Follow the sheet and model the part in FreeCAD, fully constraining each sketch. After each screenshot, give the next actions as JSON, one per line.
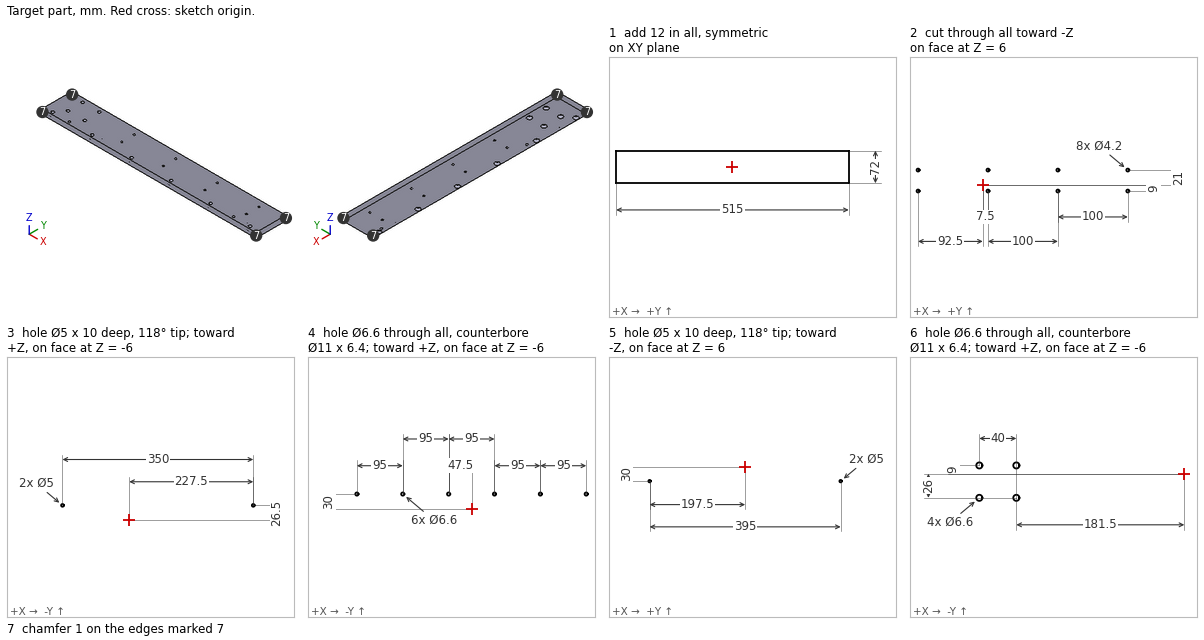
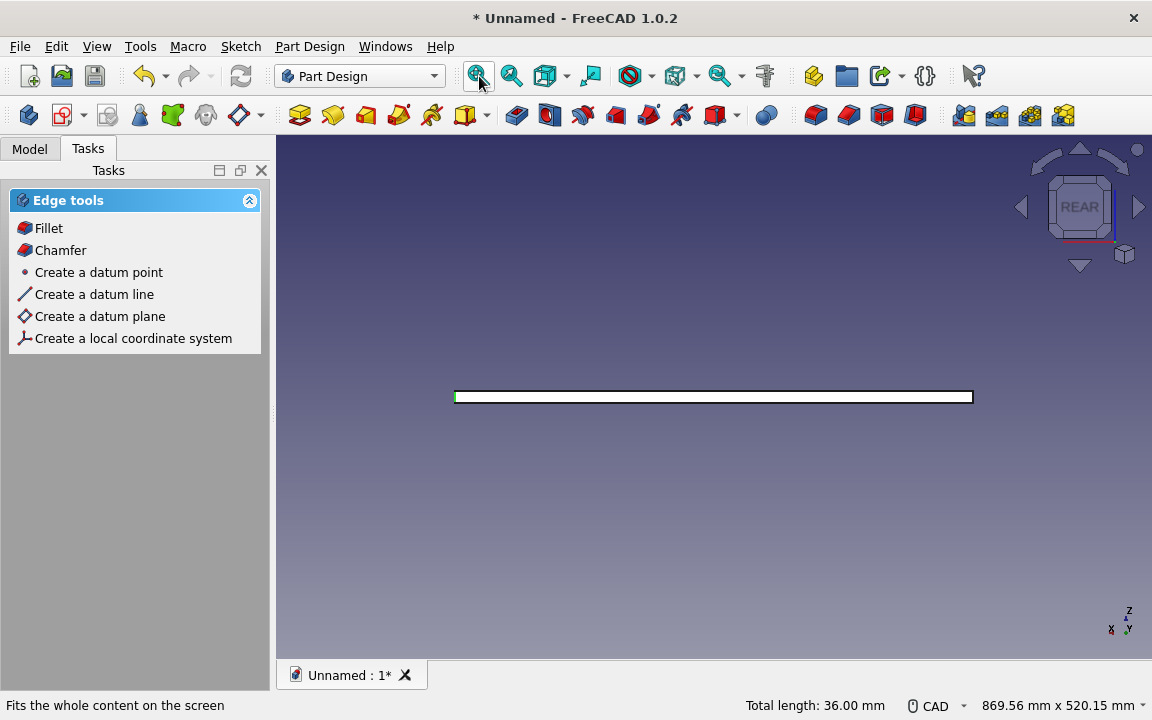
{"action": "left_click", "coordinate": [973, 396], "text": "ctrl"}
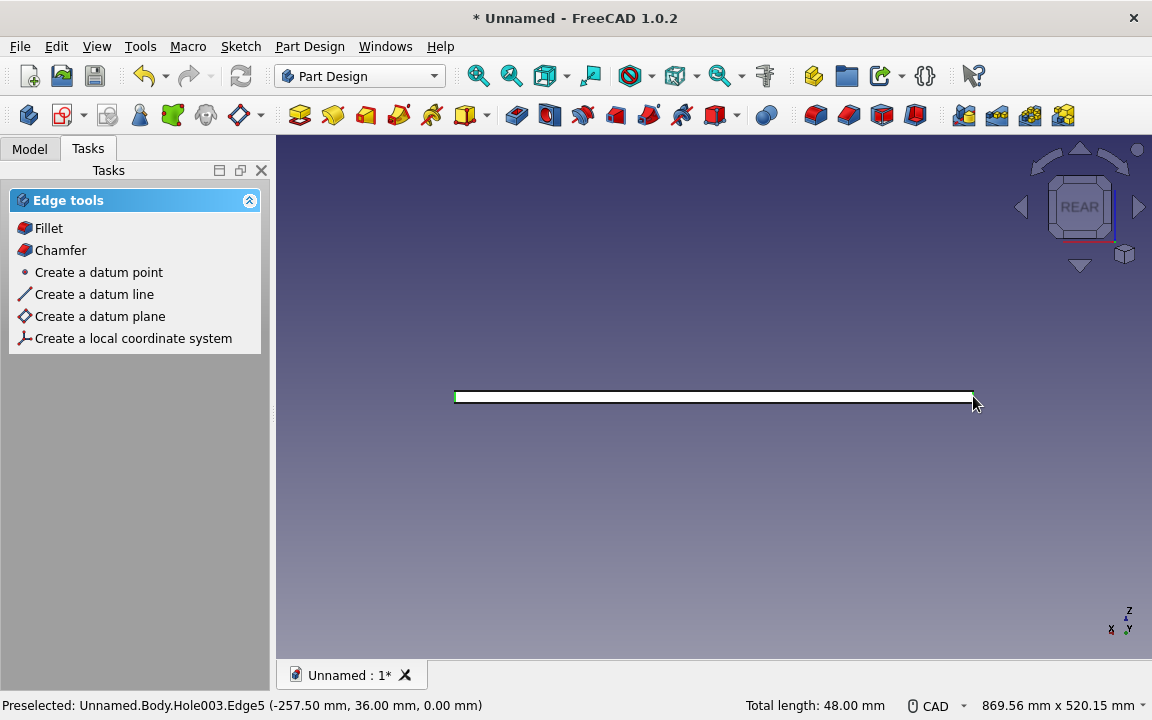
{"action": "left_click", "coordinate": [849, 116]}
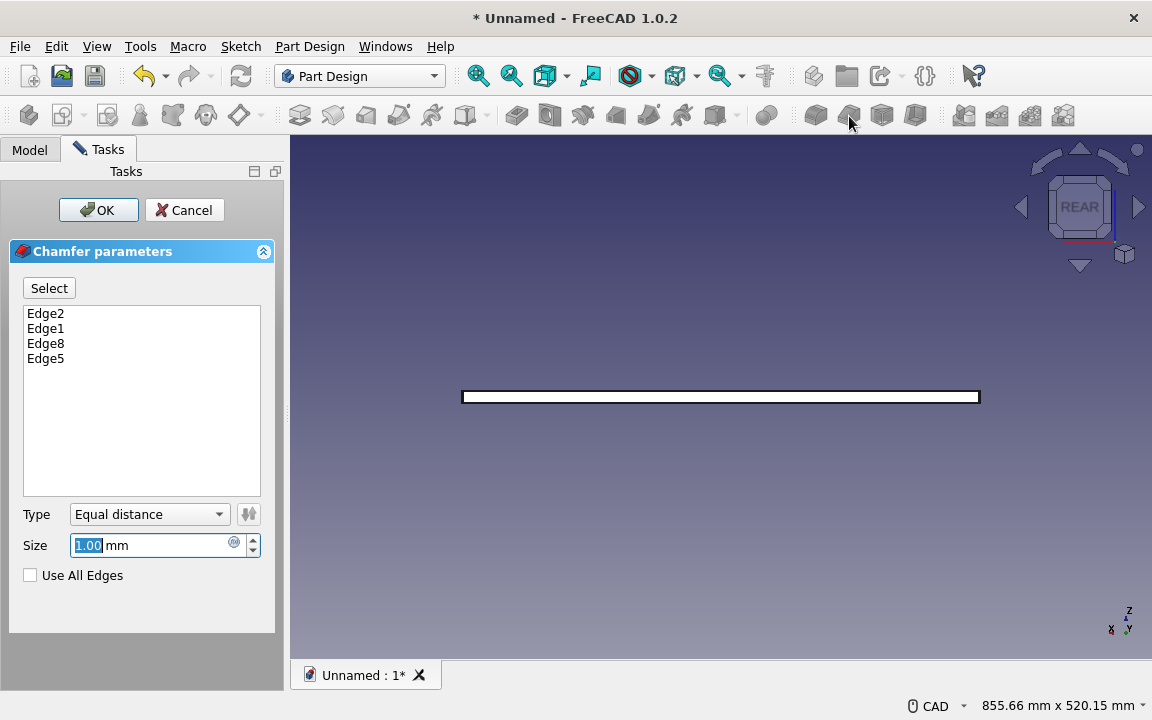
{"action": "type", "text": "1"}
{"action": "key", "text": "Tab"}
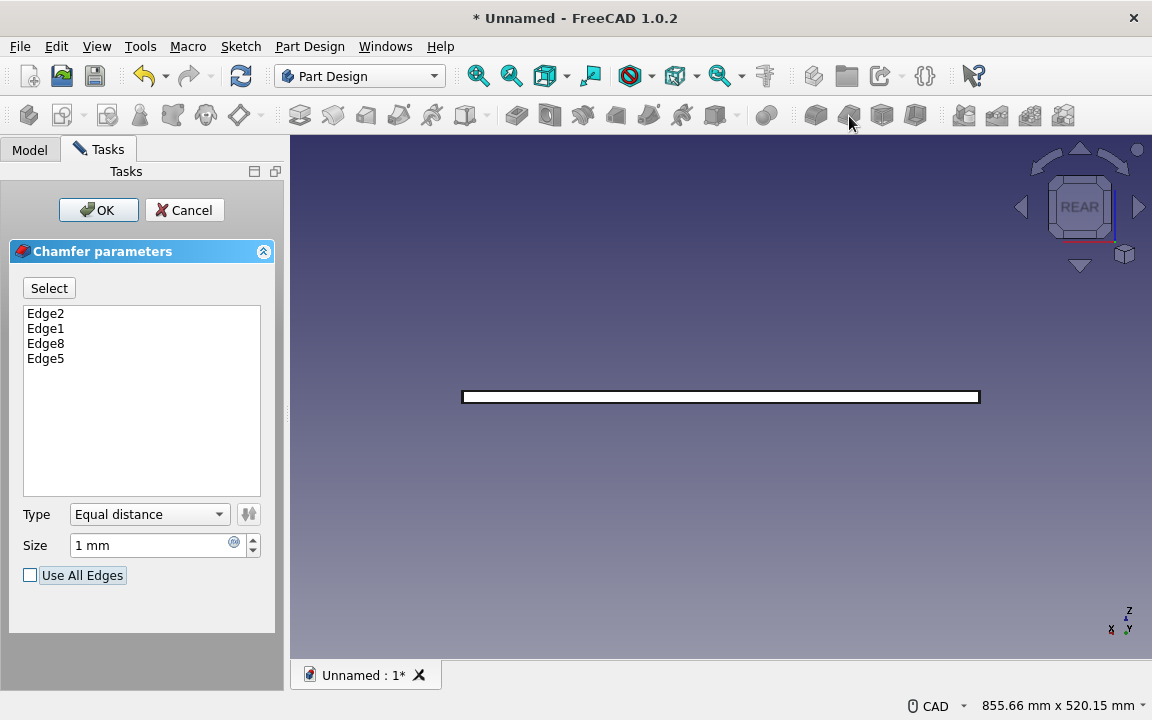
{"action": "left_click", "coordinate": [99, 210]}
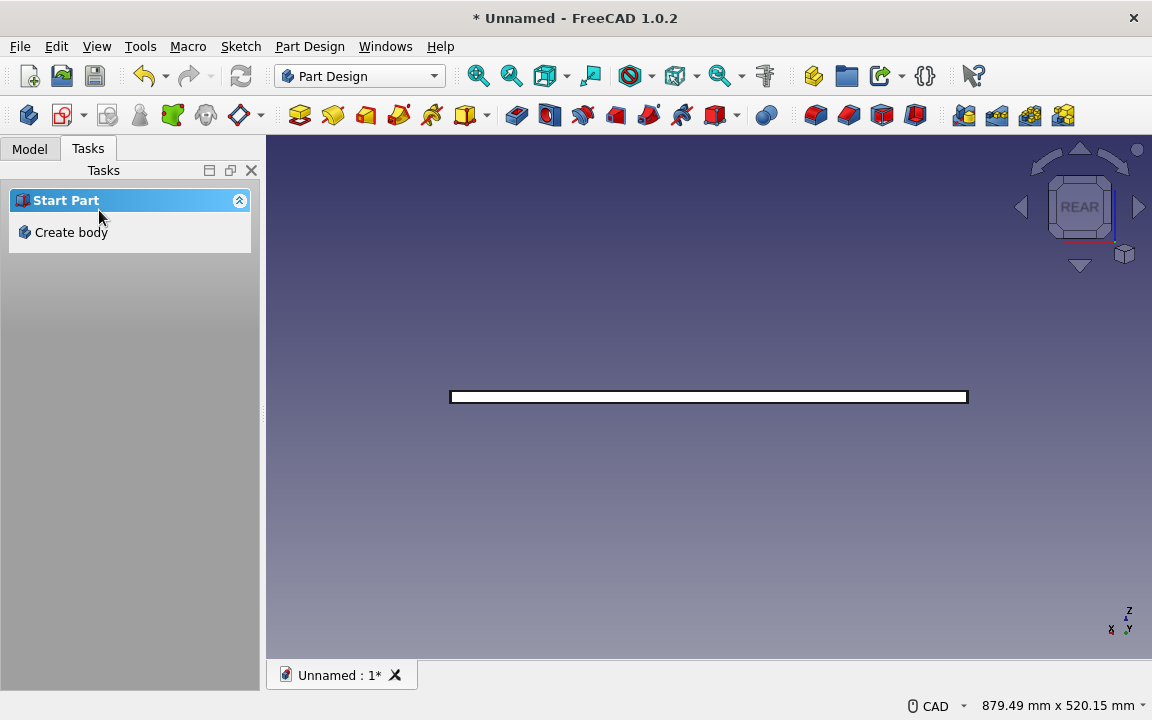
{"action": "key", "text": "0"}